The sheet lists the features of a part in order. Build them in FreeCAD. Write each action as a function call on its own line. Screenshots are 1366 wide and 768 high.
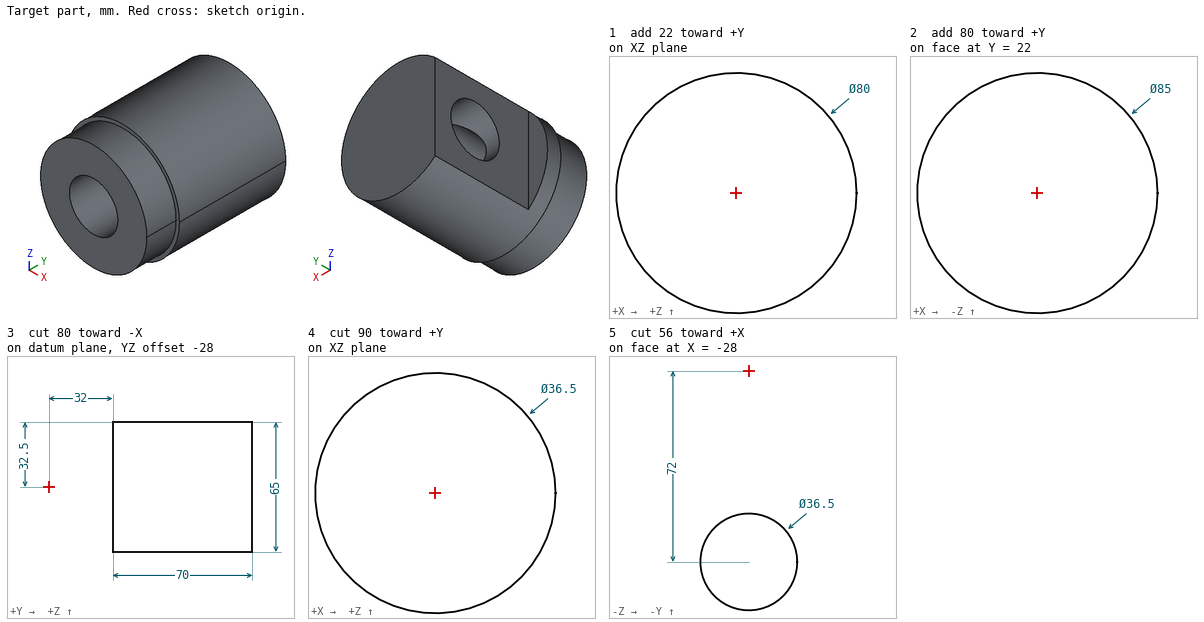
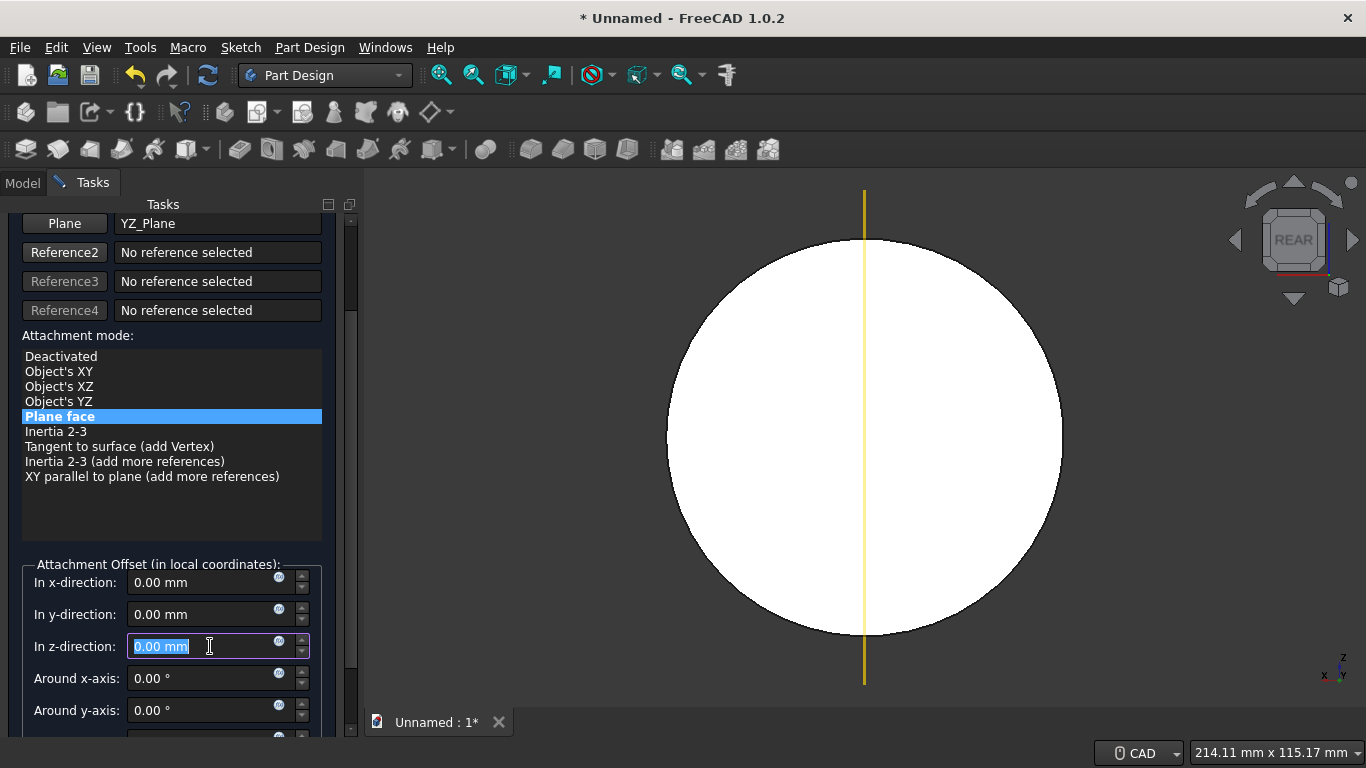
text(-28)
key(Tab)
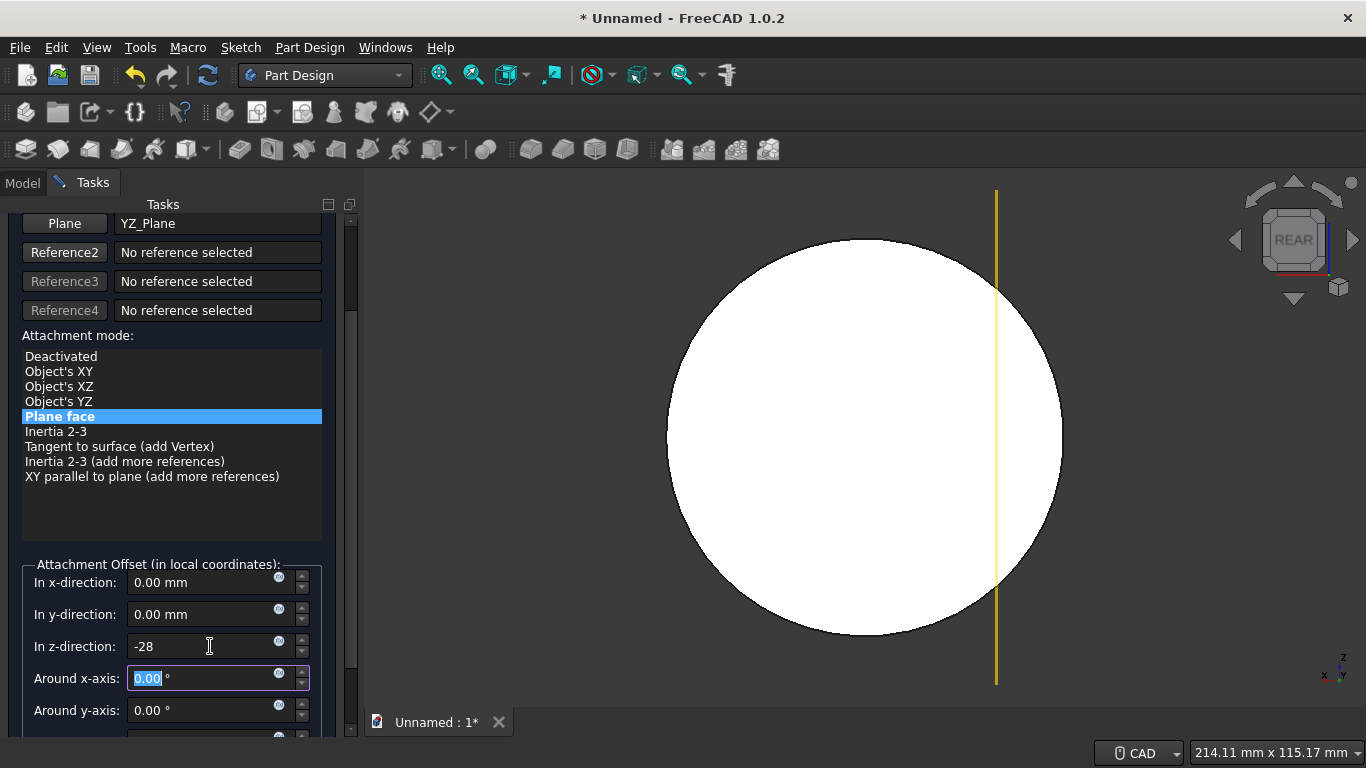
scroll(351, 475, up, 3)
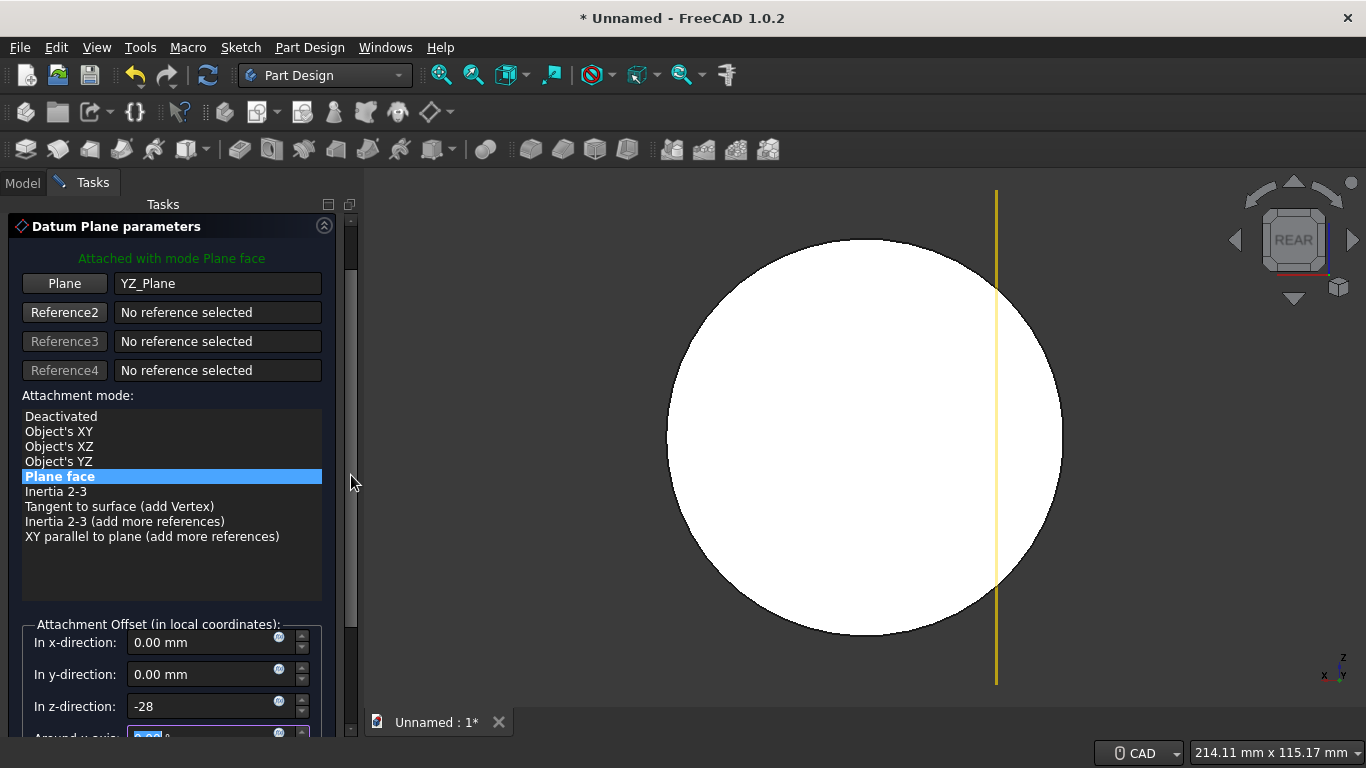
click(124, 243)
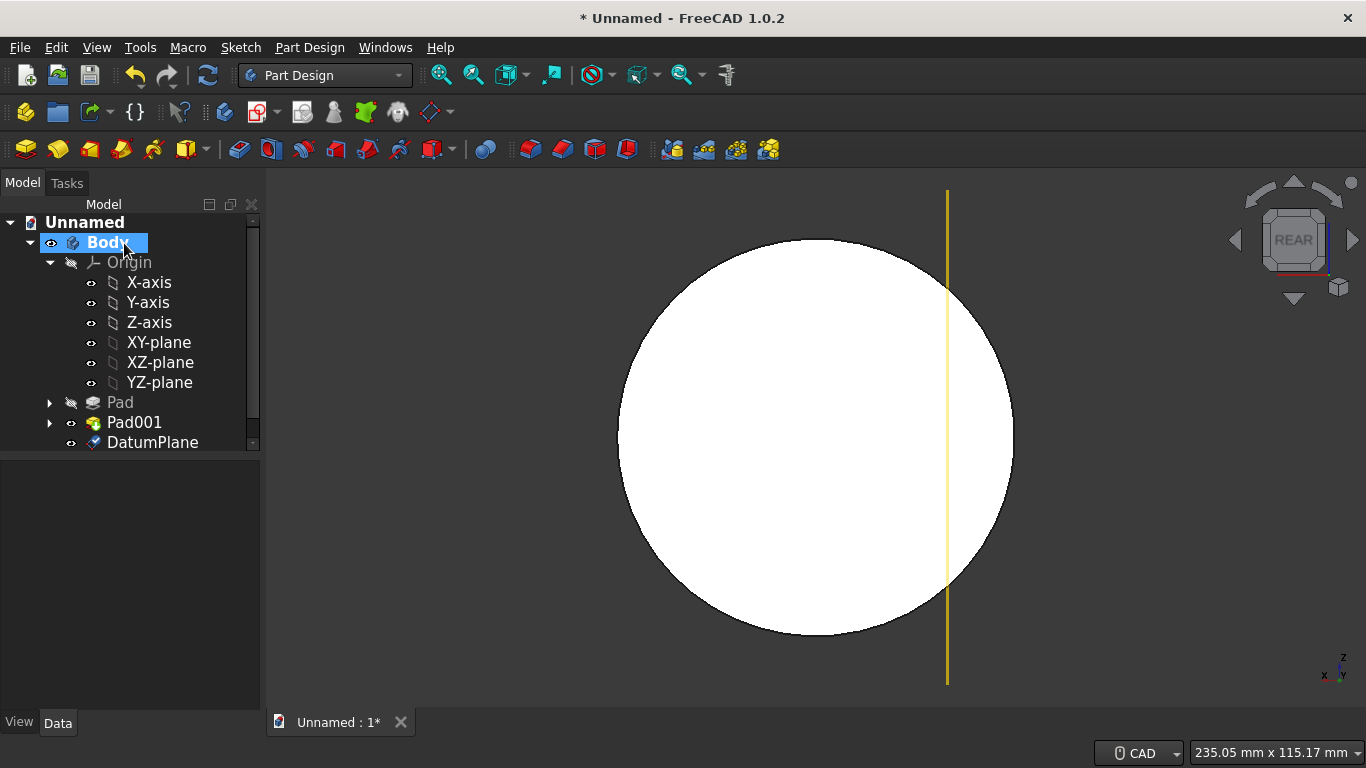
click(116, 443)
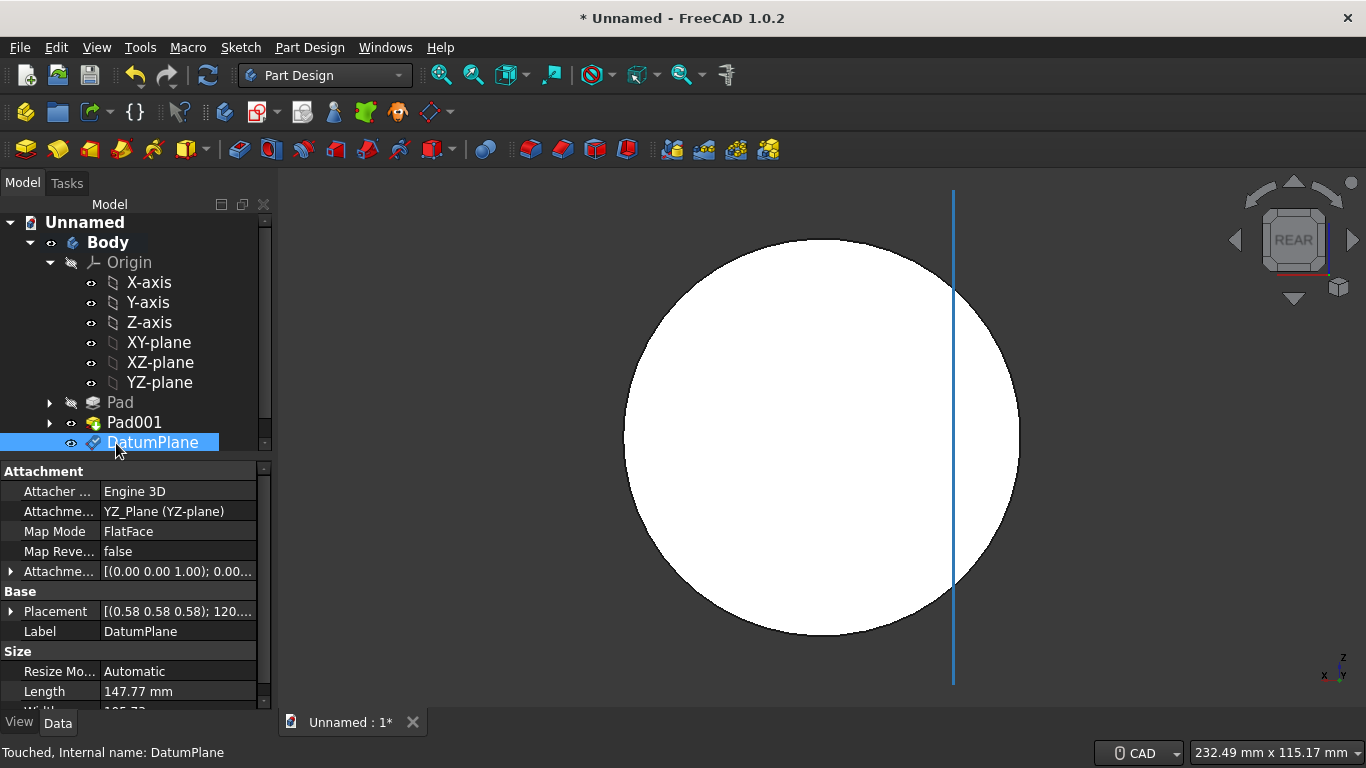
click(258, 112)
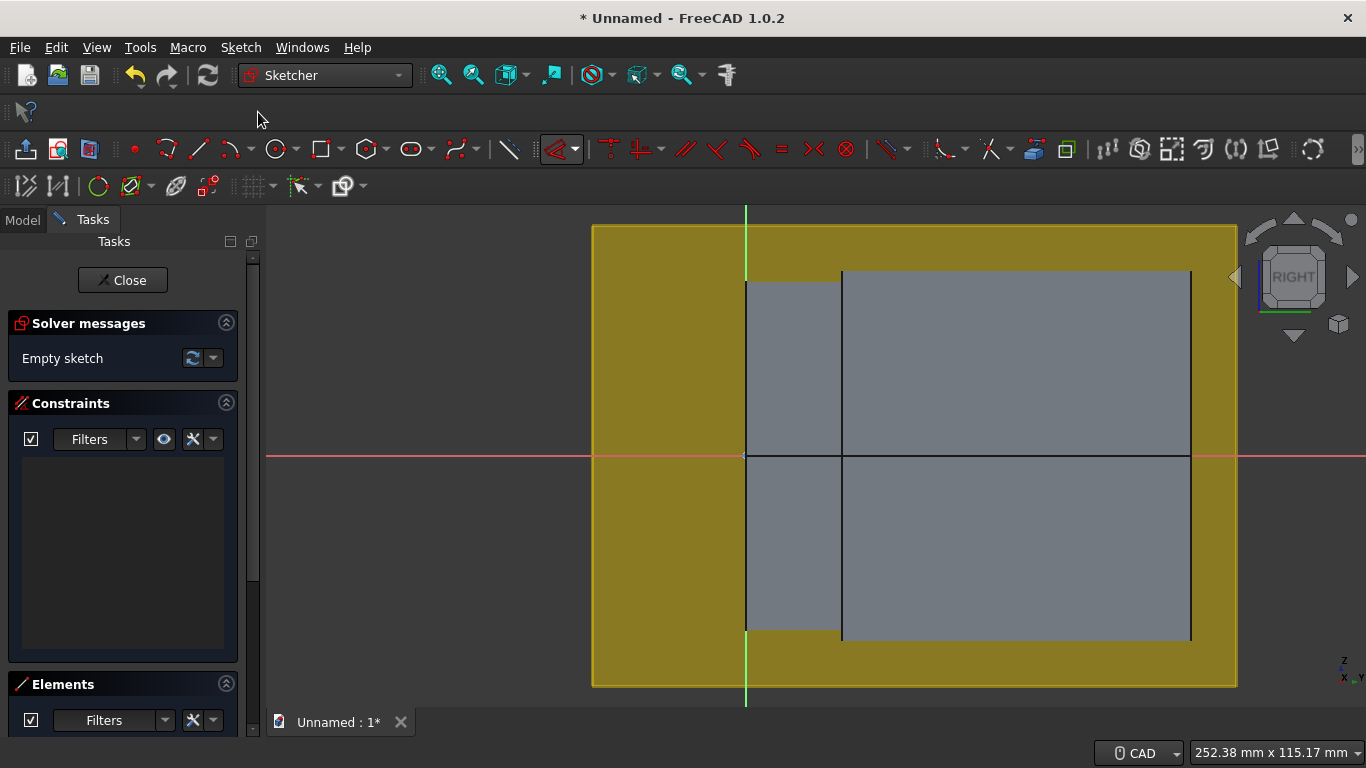
click(90, 150)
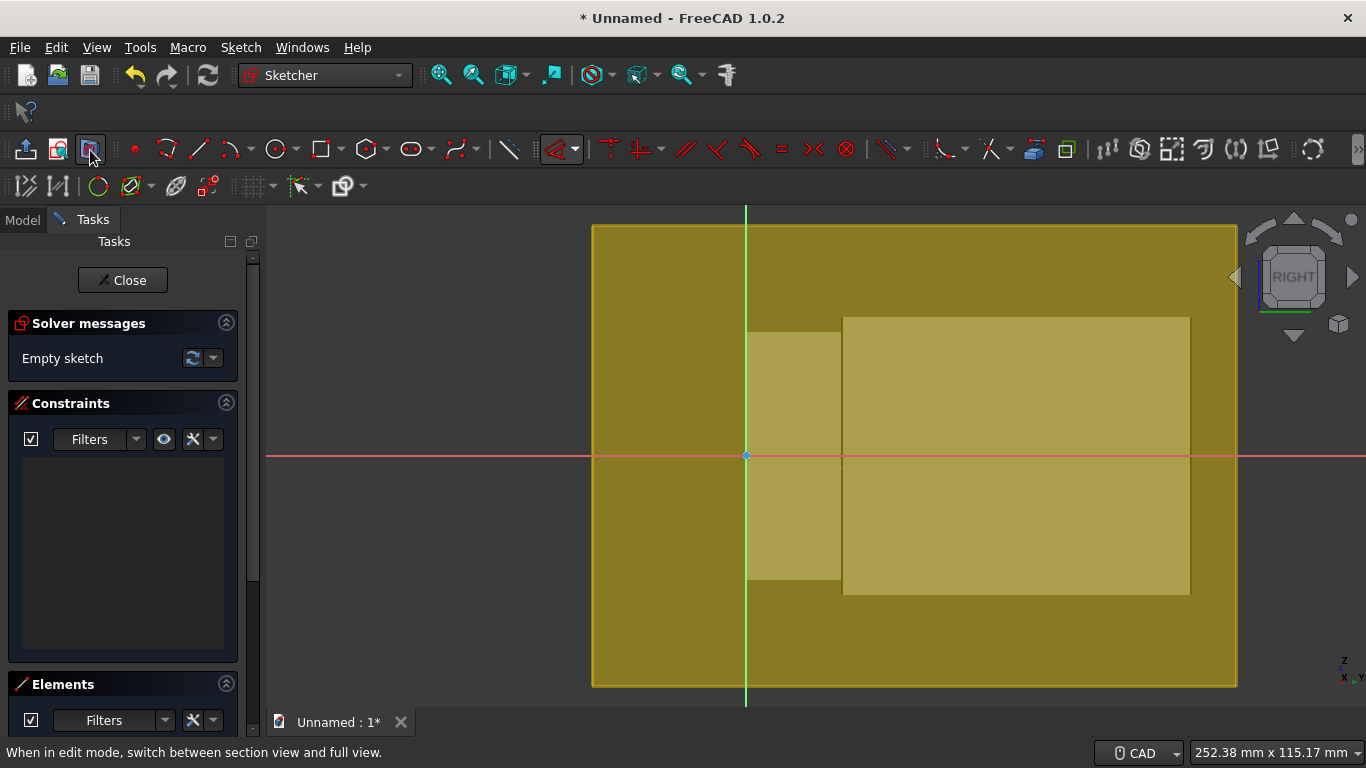
scroll(294, 456, down, 1)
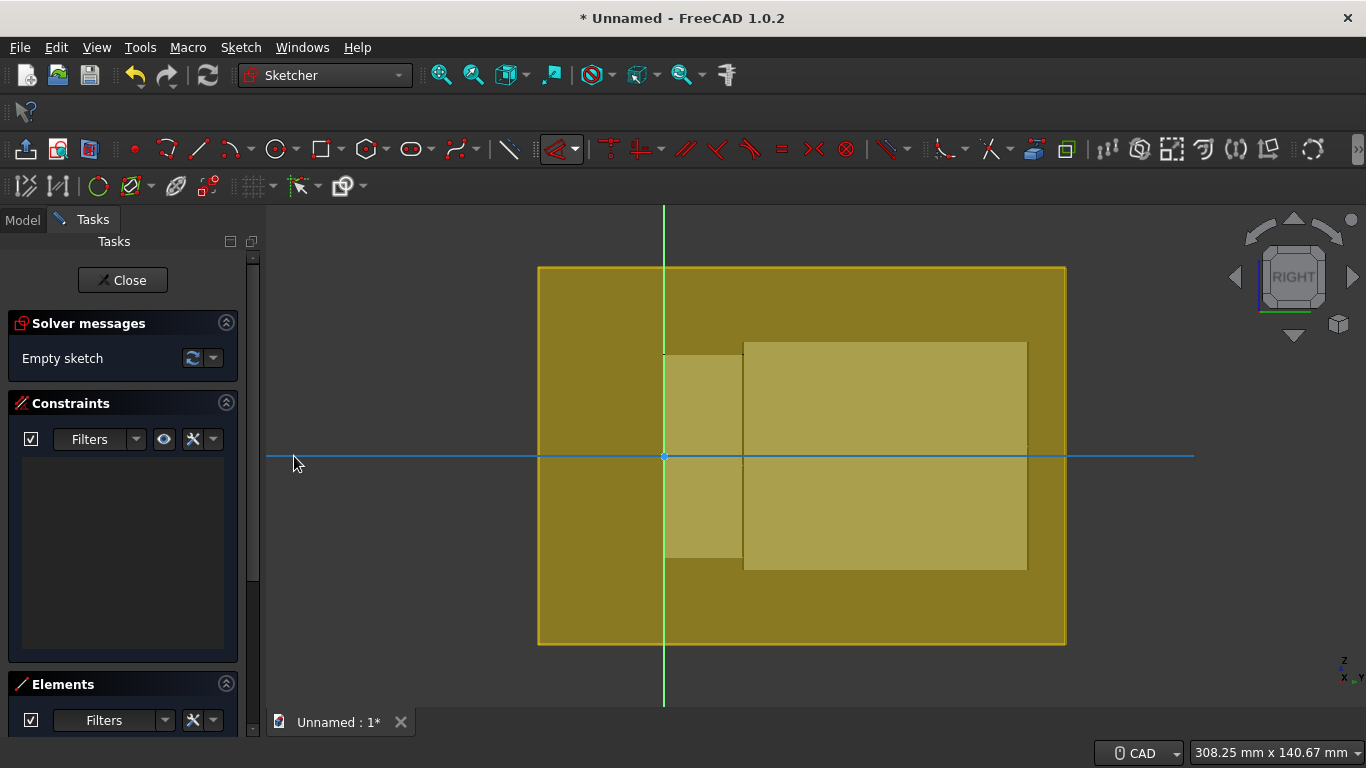
scroll(1047, 456, up, 2)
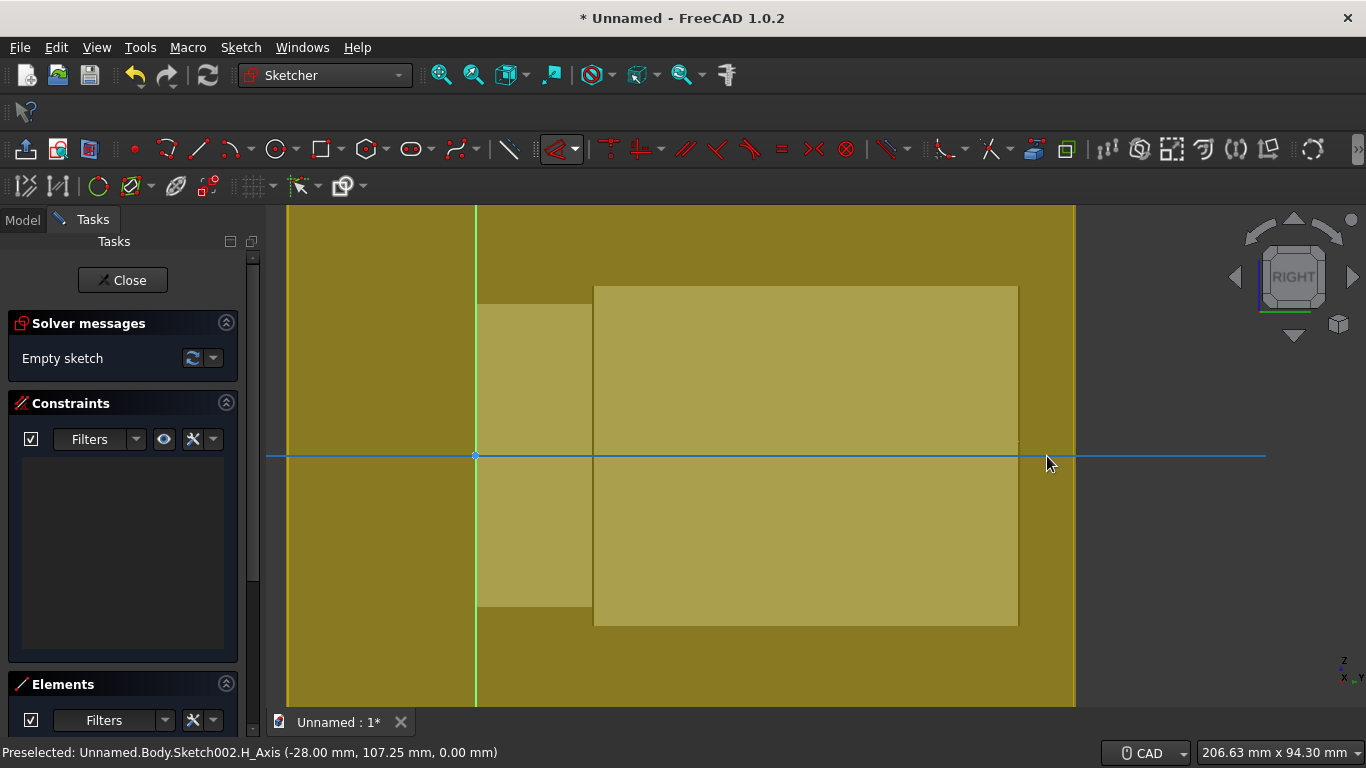
click(322, 150)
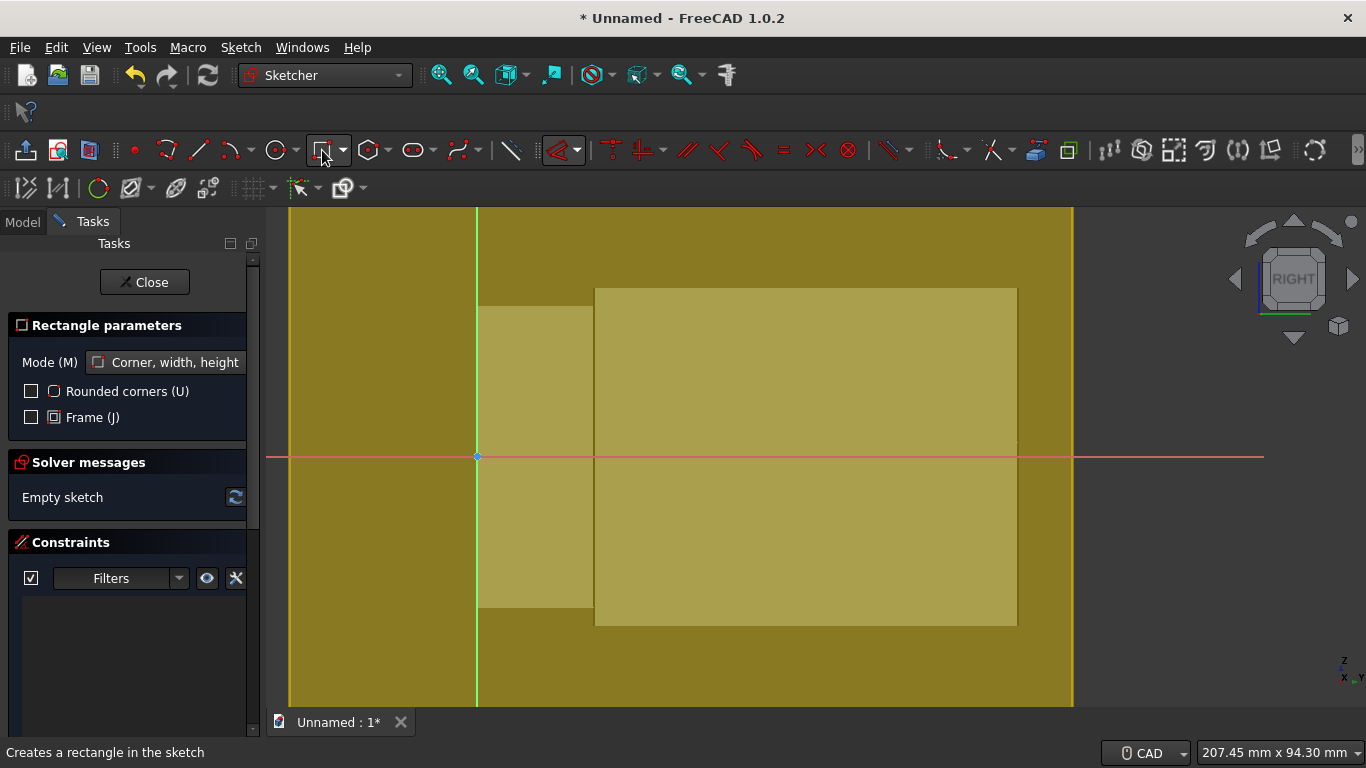
click(647, 285)
move(1018, 629)